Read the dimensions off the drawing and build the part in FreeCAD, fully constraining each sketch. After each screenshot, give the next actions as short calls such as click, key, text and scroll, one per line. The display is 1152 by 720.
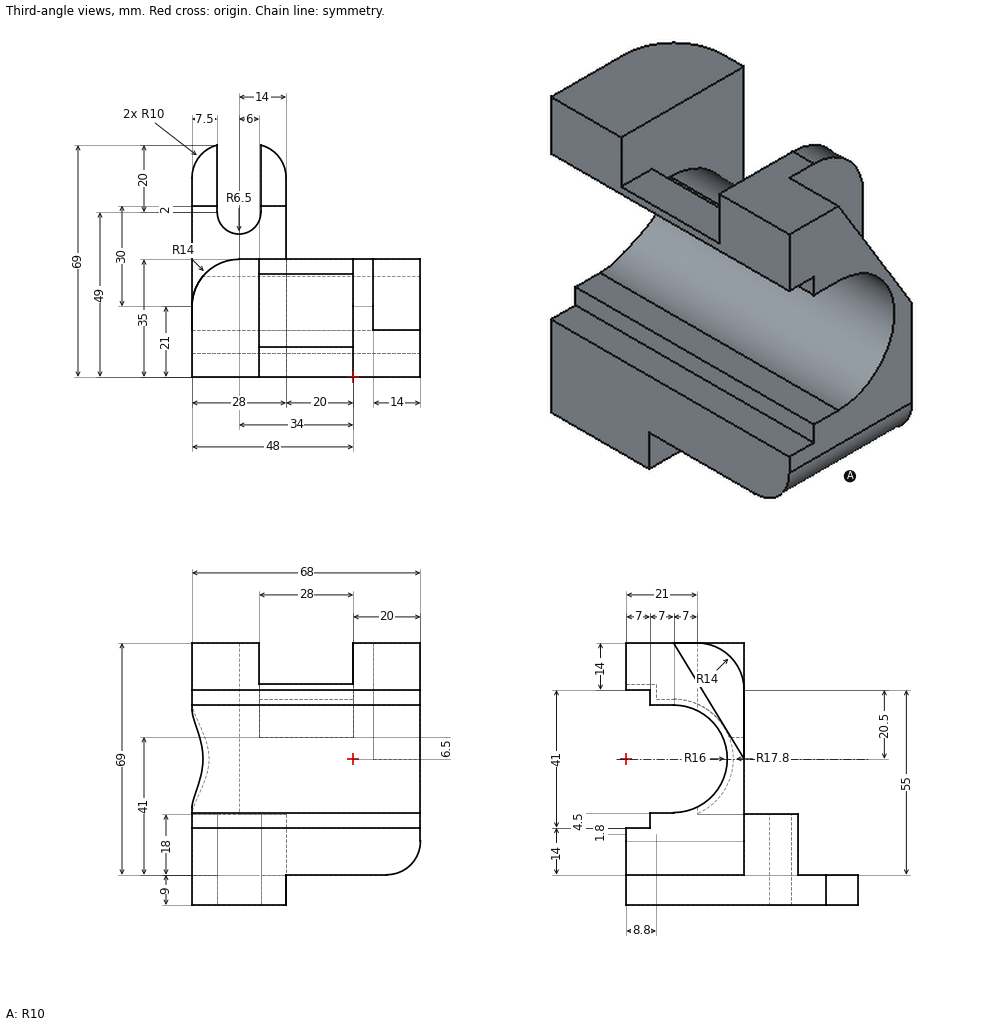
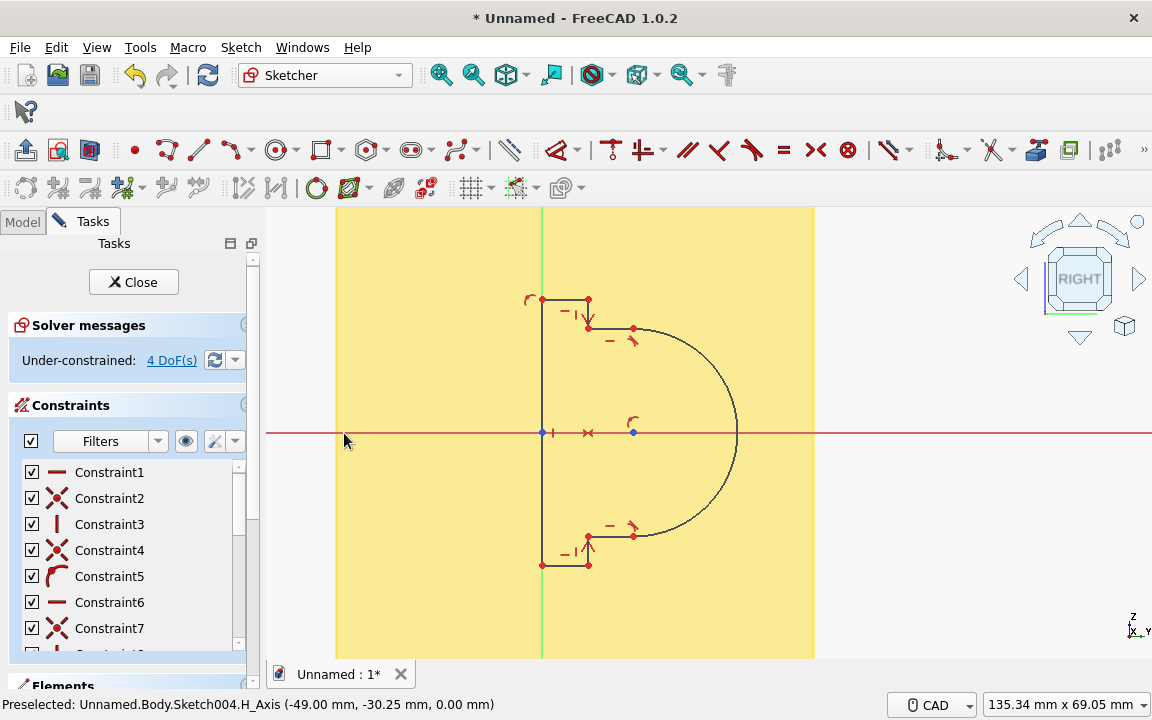
key(d)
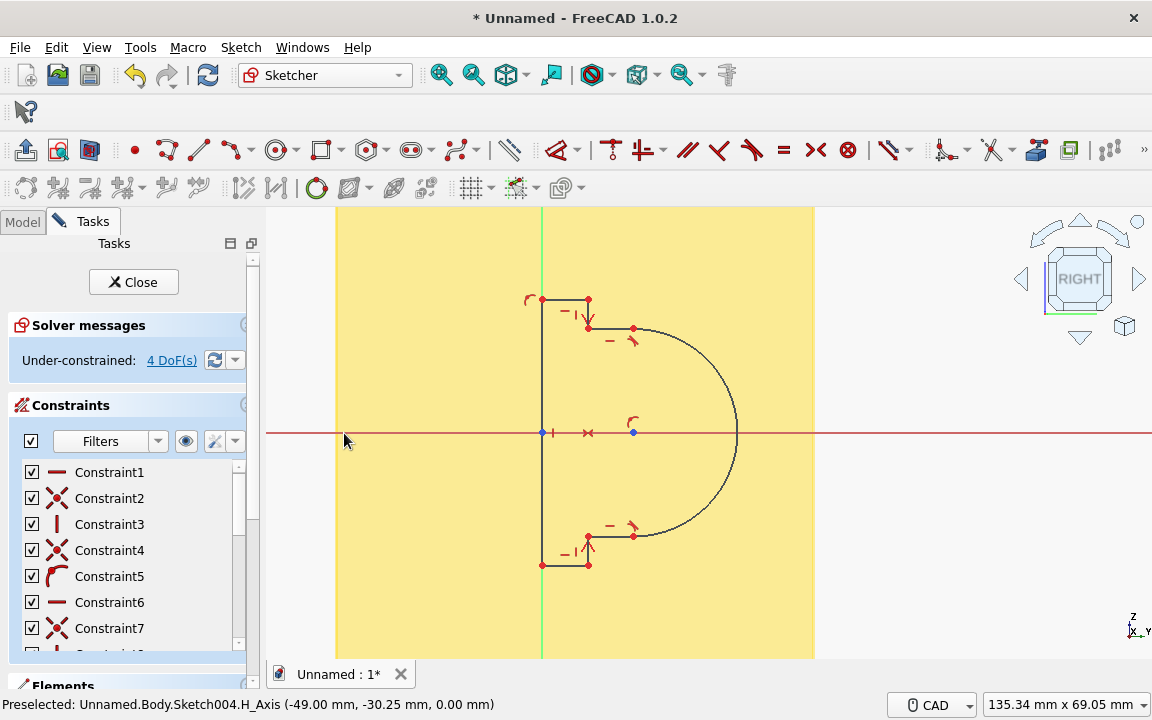
click(718, 494)
click(744, 513)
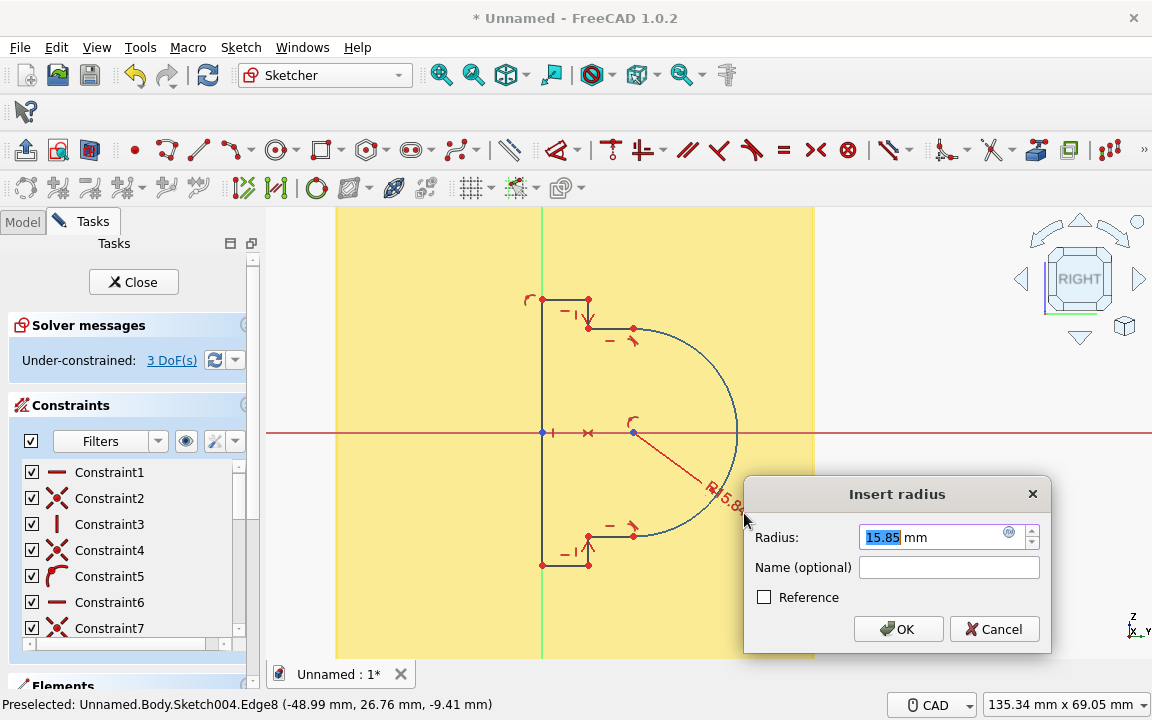
text(16)
key(Return)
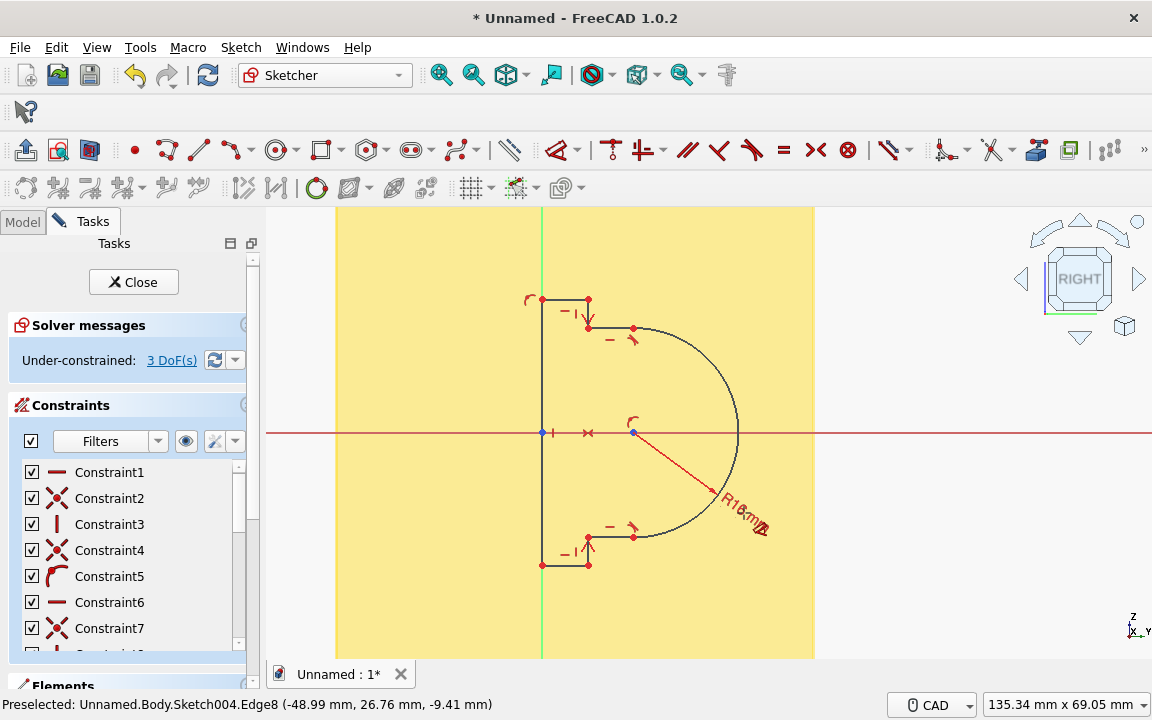
click(620, 328)
click(611, 294)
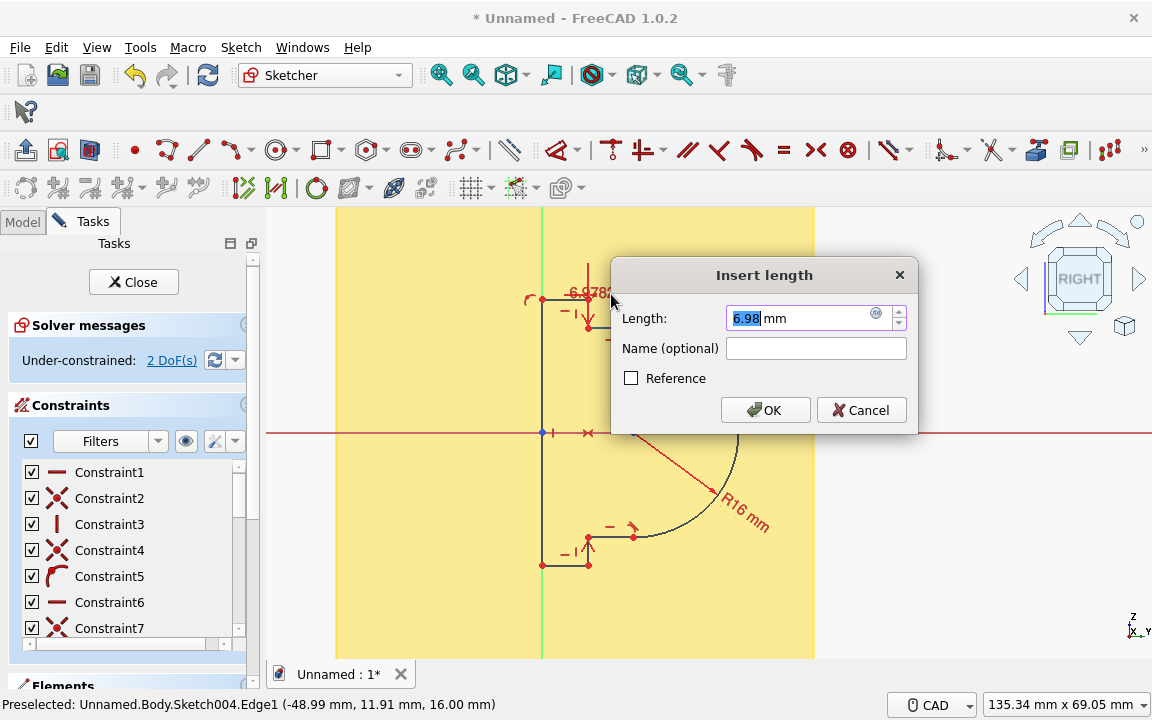
text(7)
key(Return)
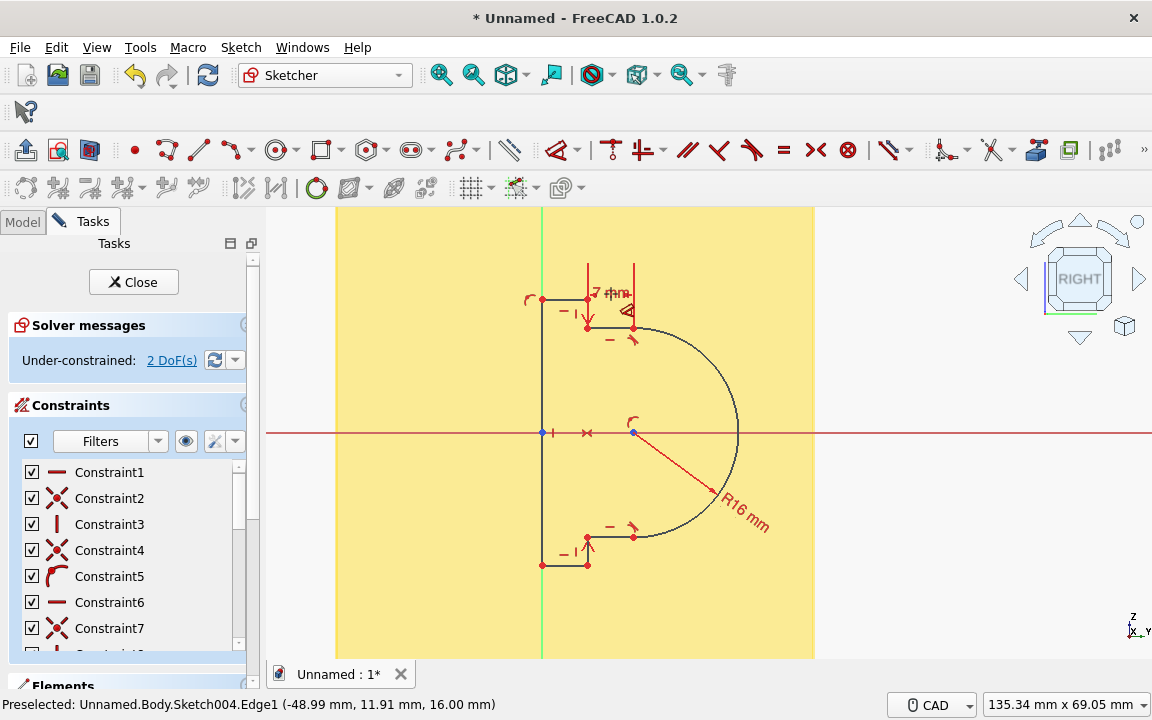
click(574, 300)
click(565, 266)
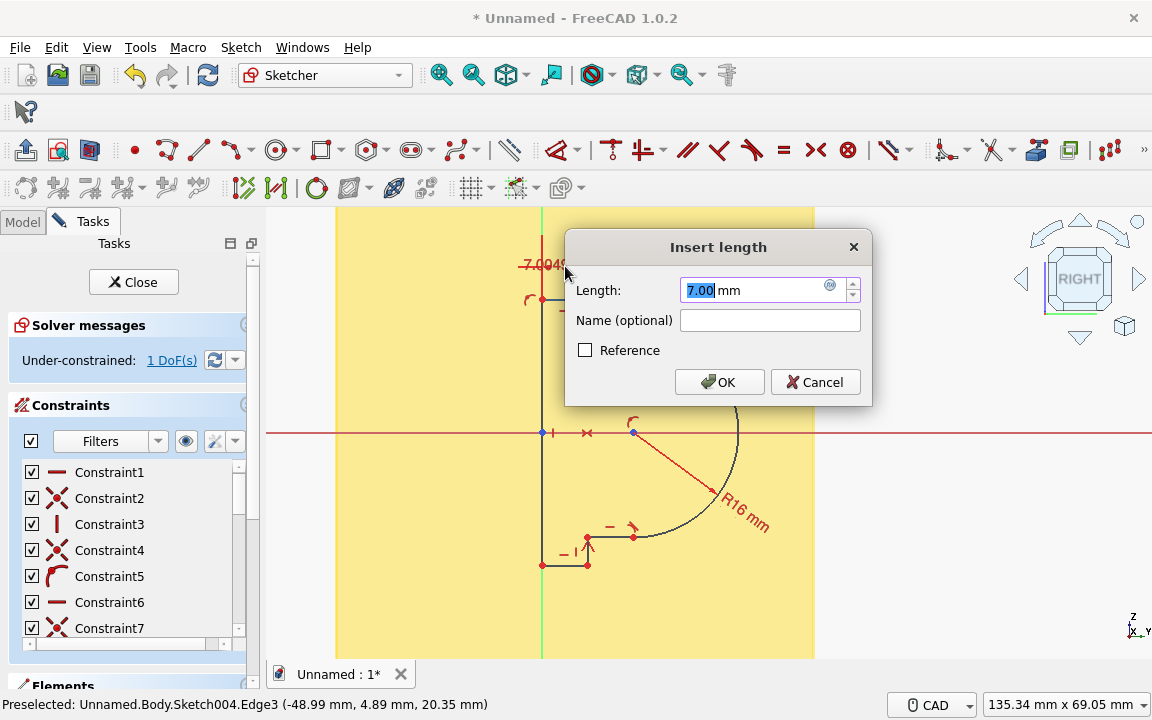
text(7)
key(Return)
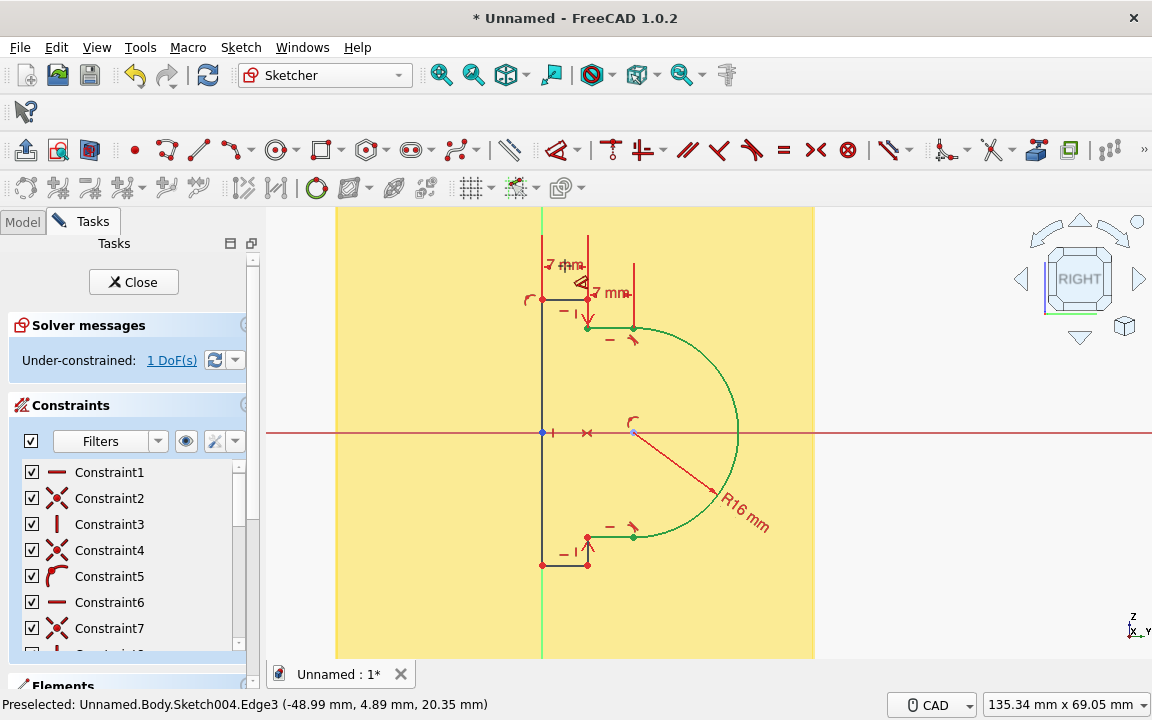
click(542, 379)
click(508, 371)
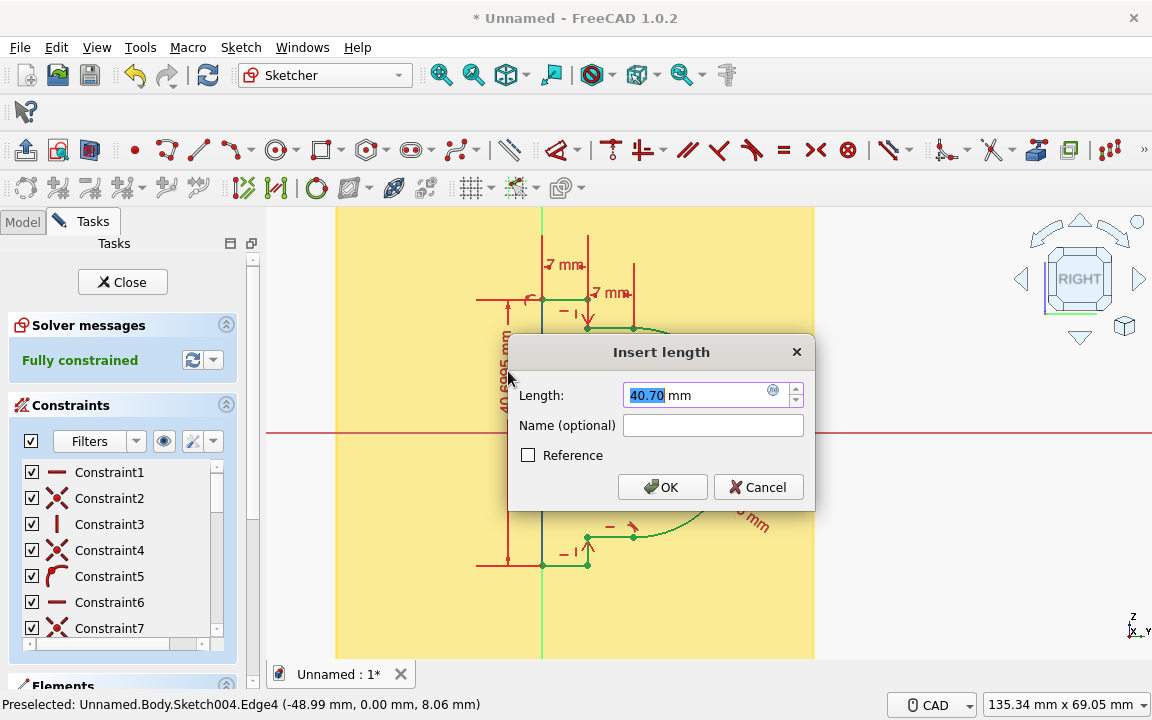
text(41)
key(Return)
key(Escape)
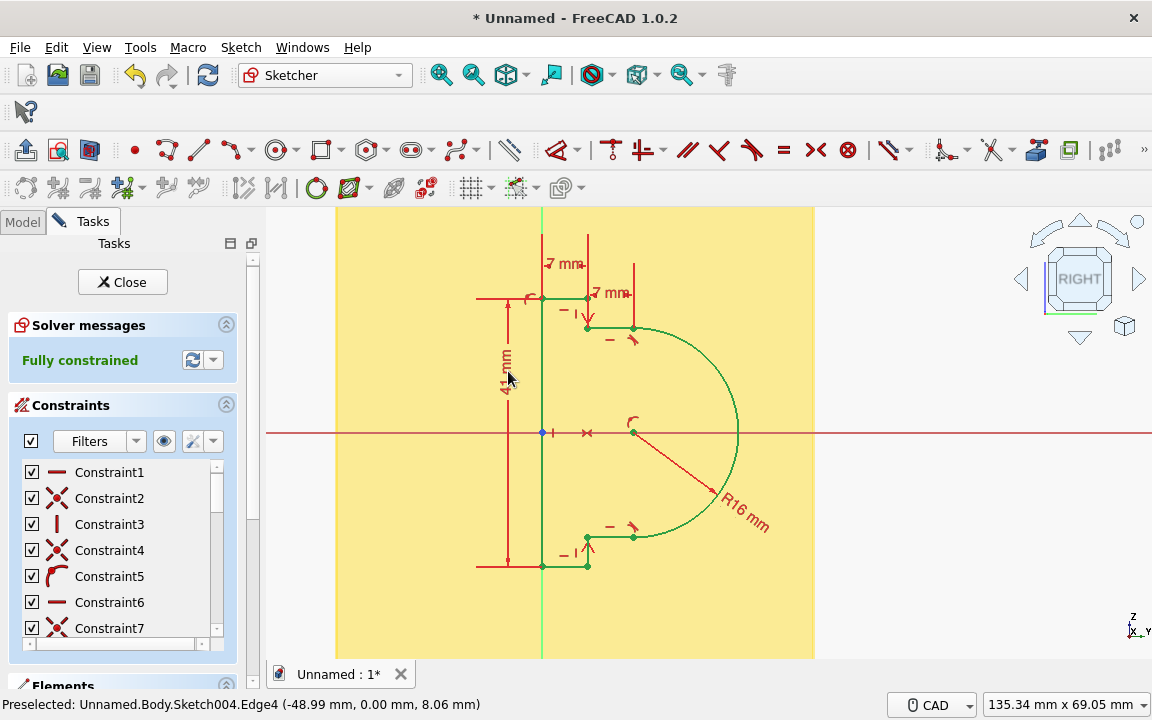
click(123, 282)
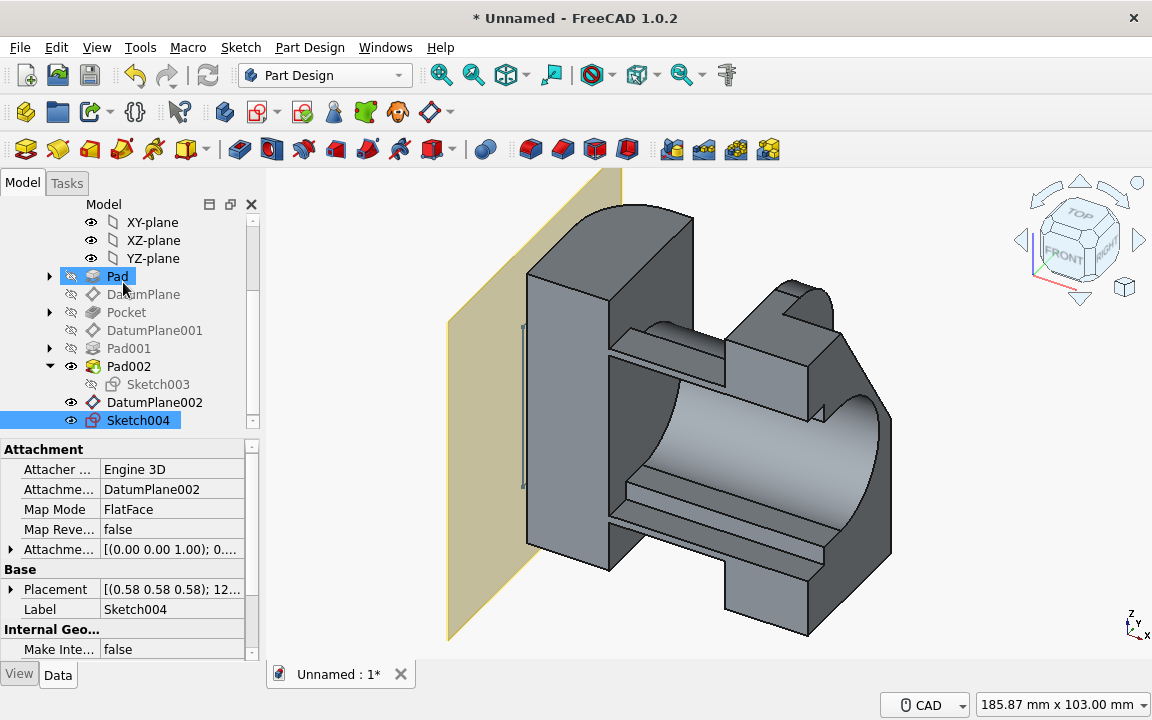
click(240, 150)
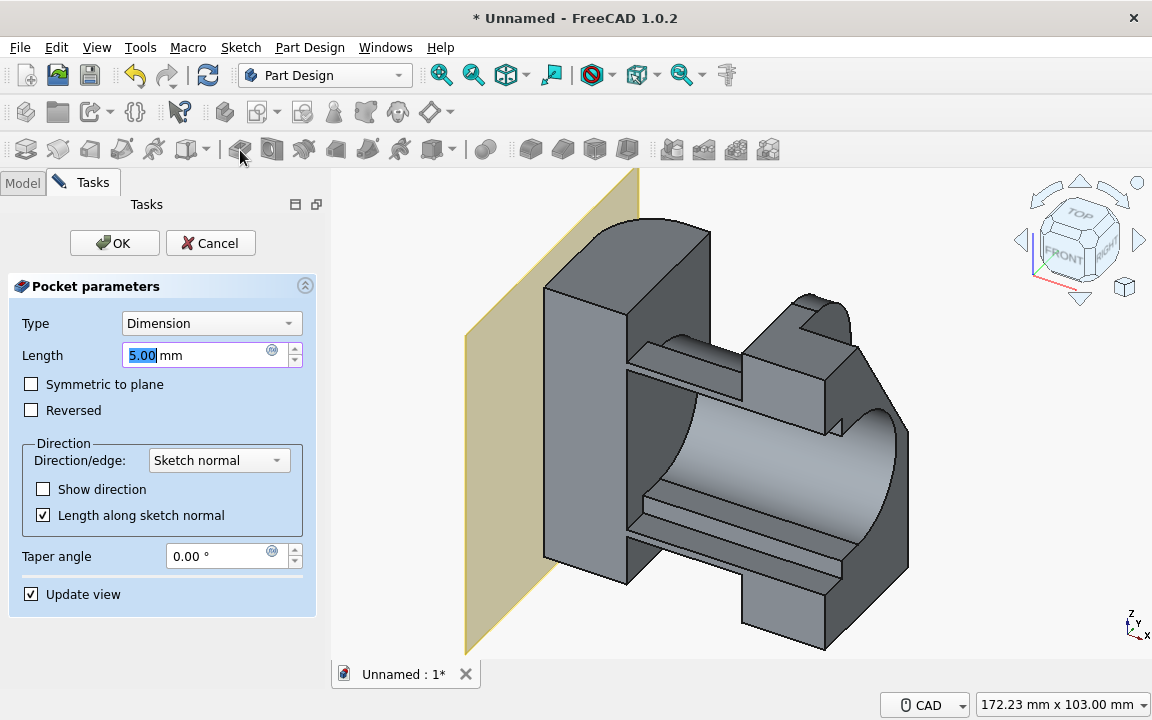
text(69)
key(Tab)